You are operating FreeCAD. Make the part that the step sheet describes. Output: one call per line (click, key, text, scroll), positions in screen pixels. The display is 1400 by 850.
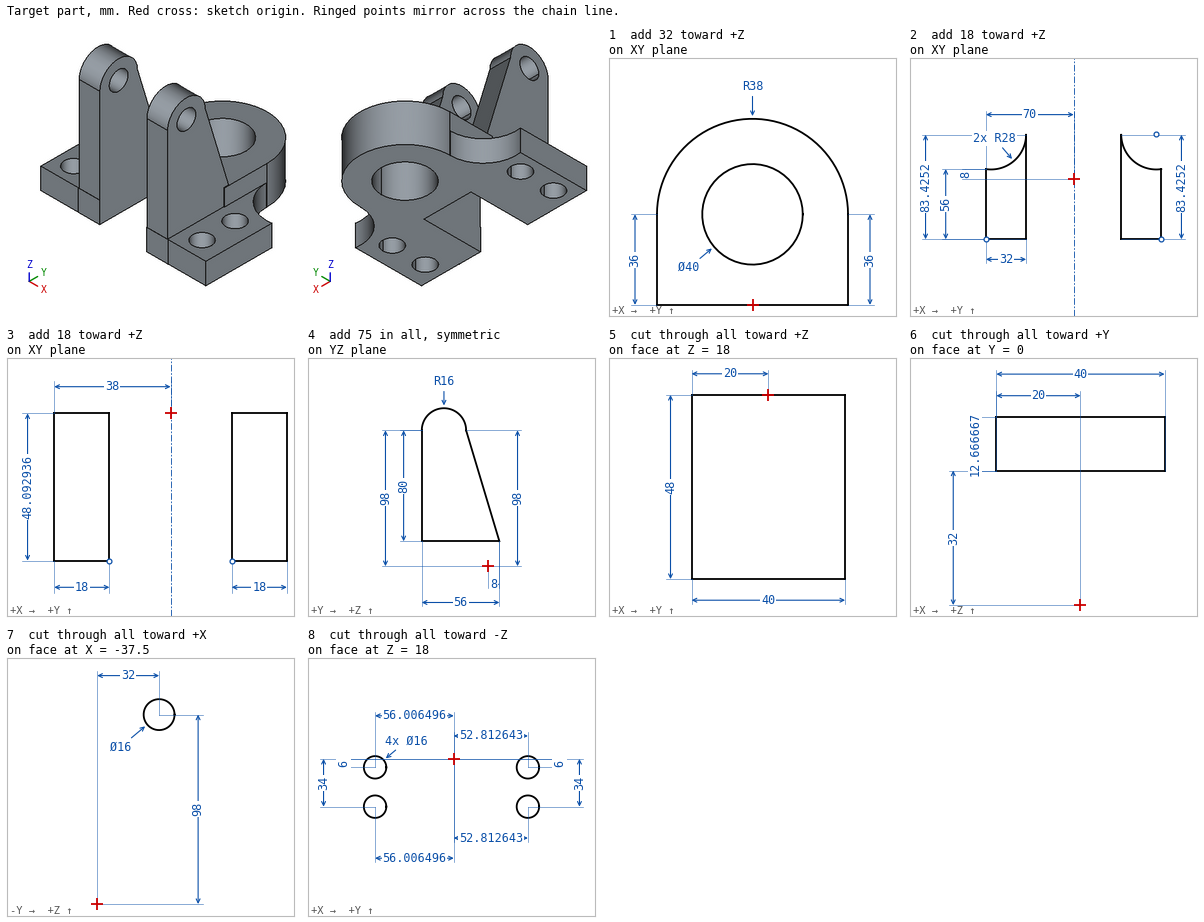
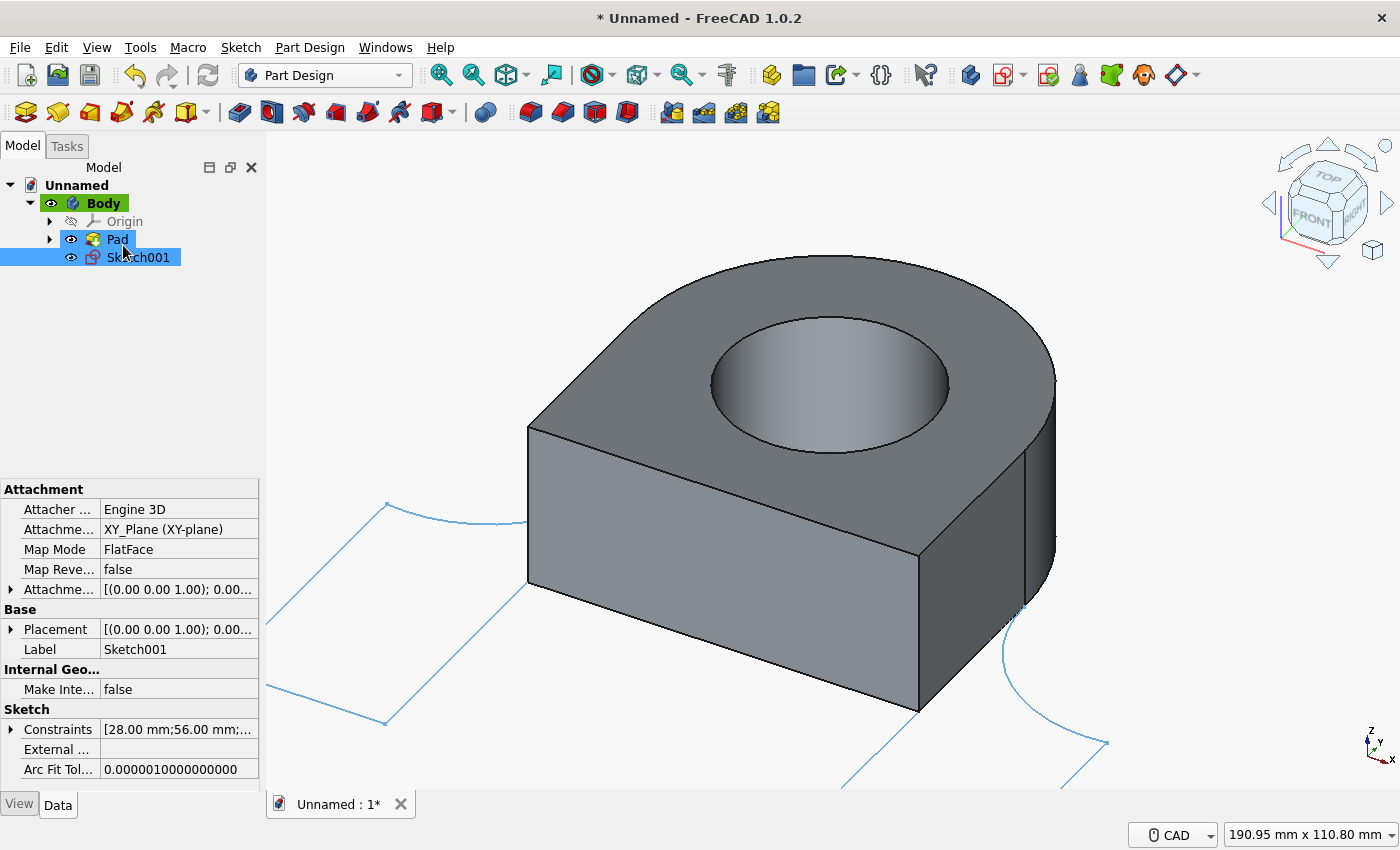
click(26, 112)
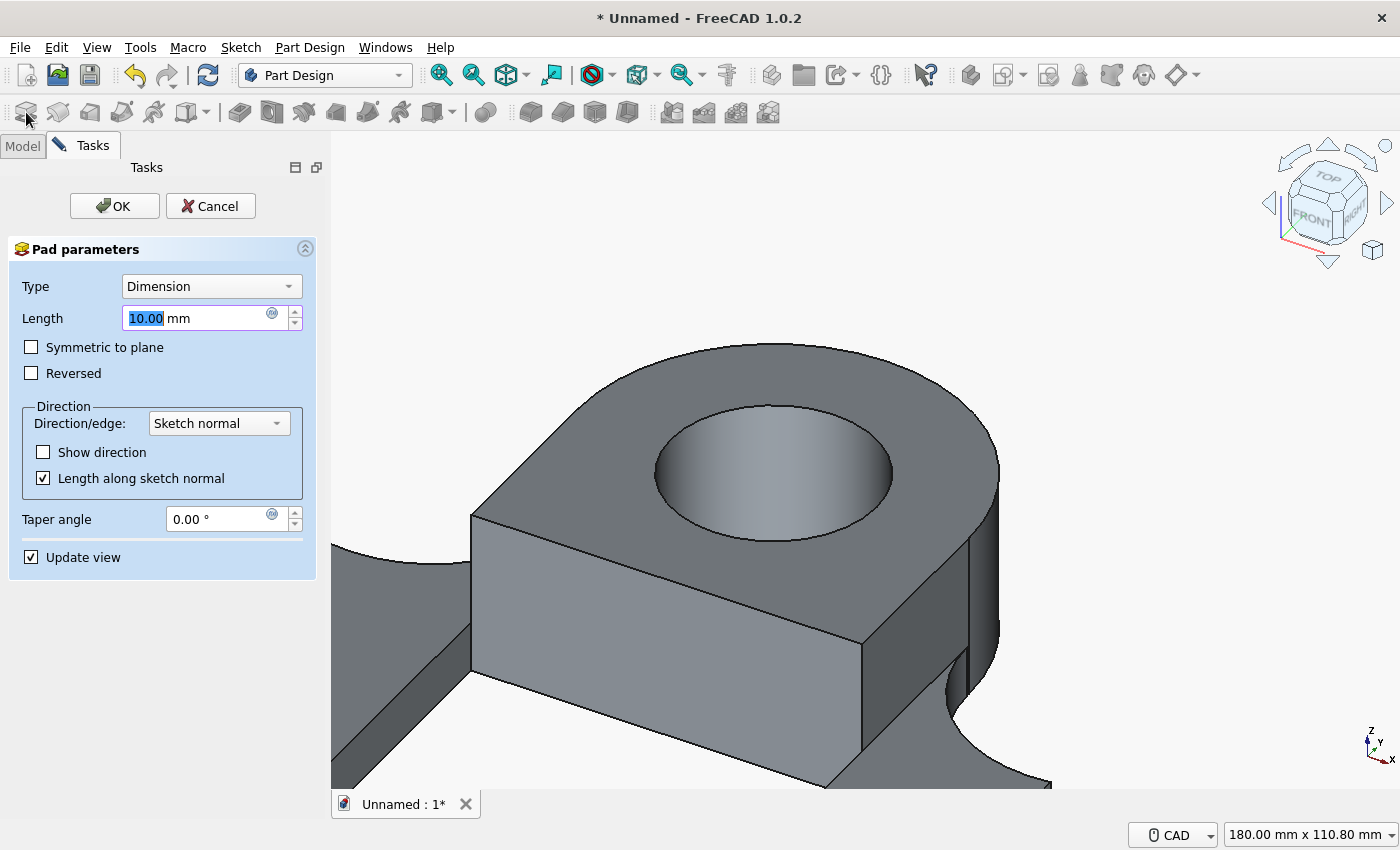
text(18)
key(Tab)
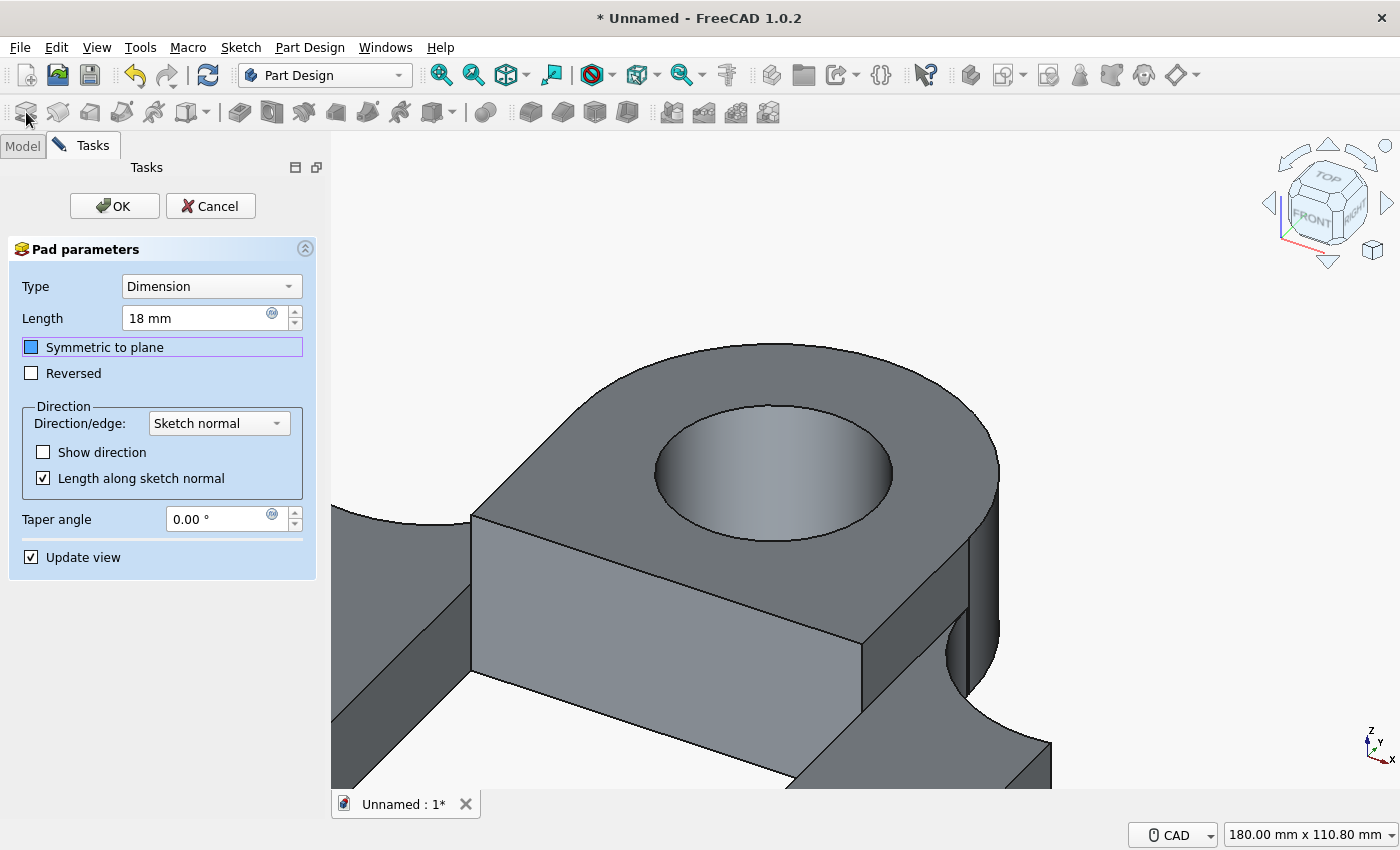
click(115, 206)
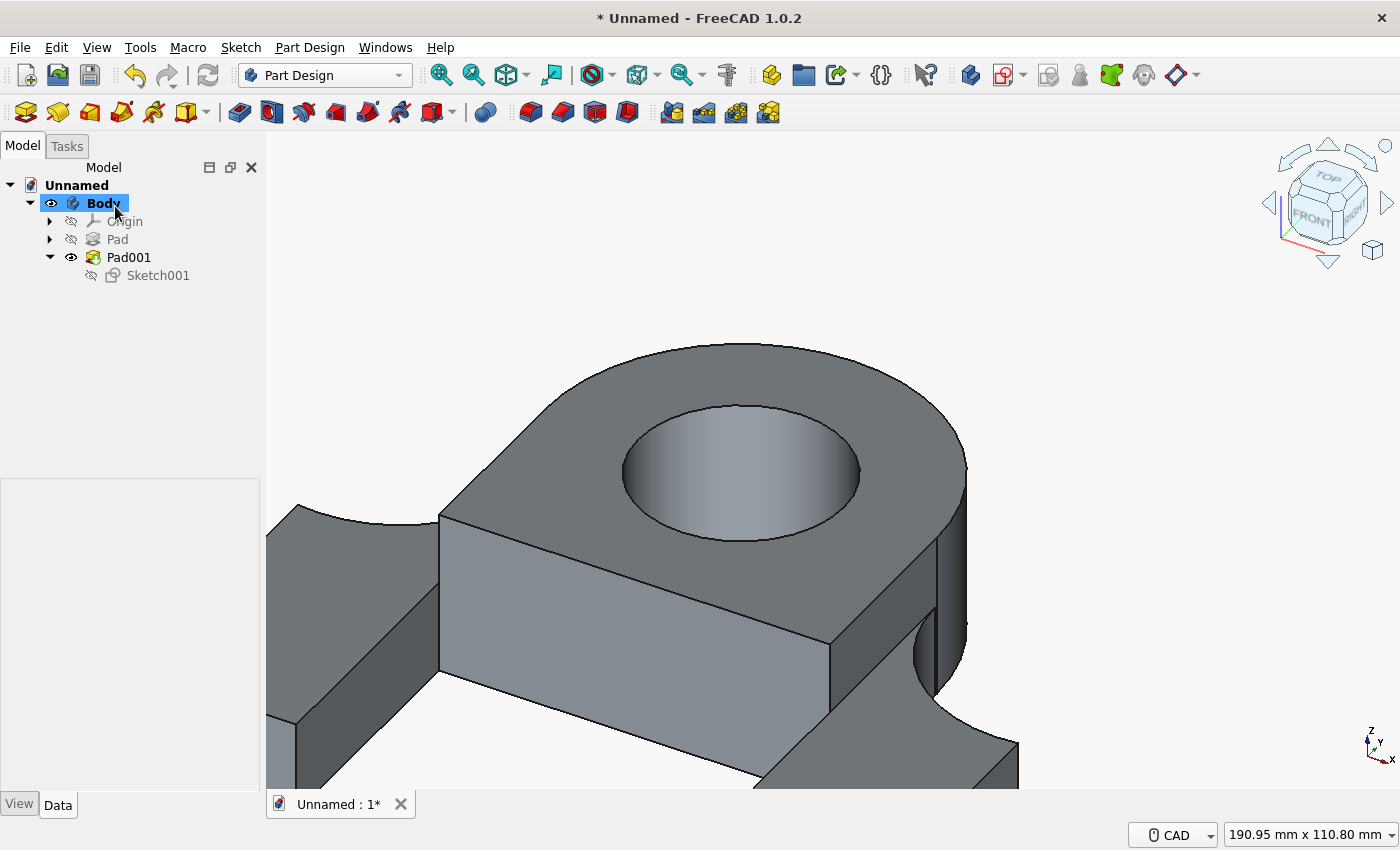
click(442, 76)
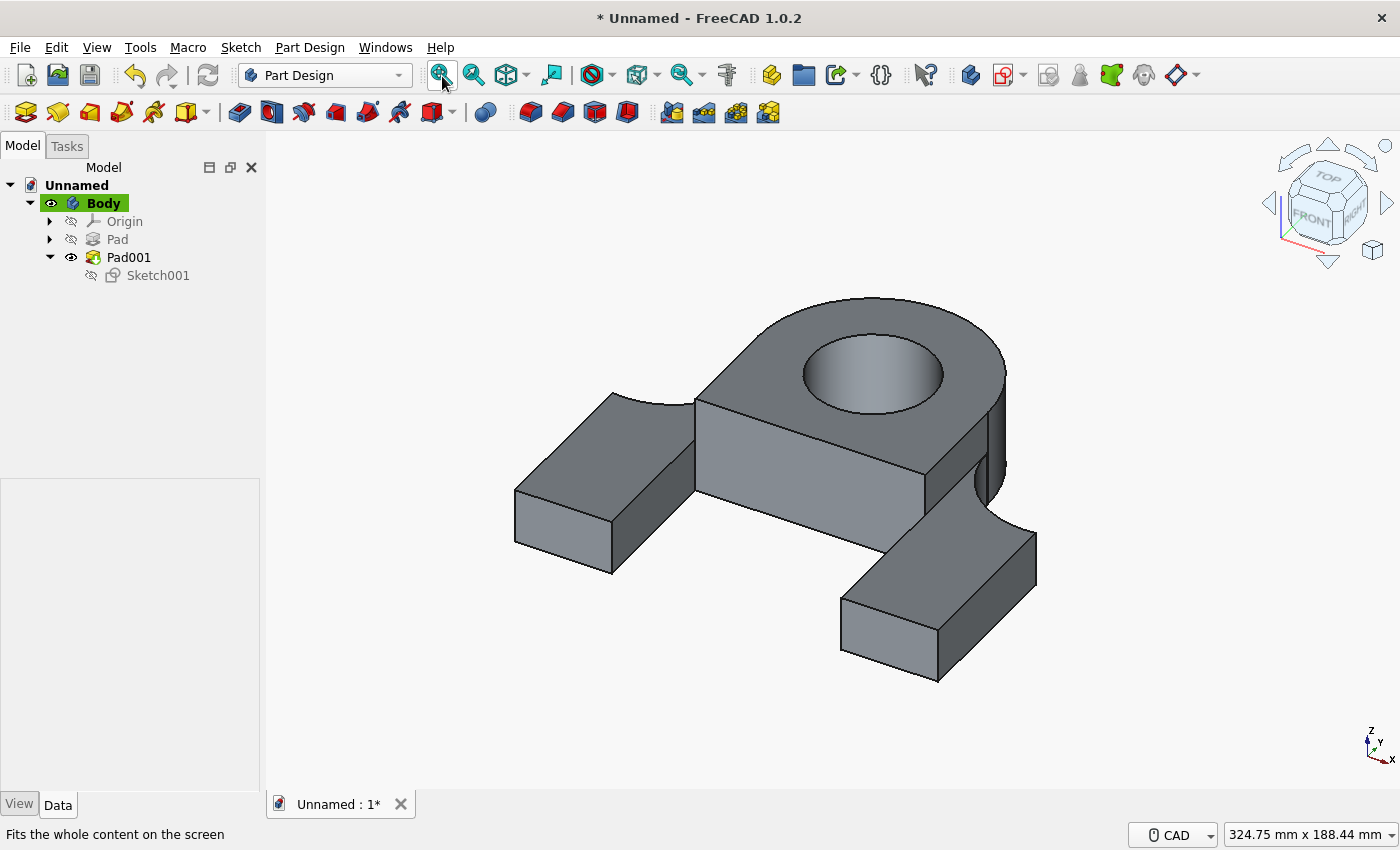
click(1004, 76)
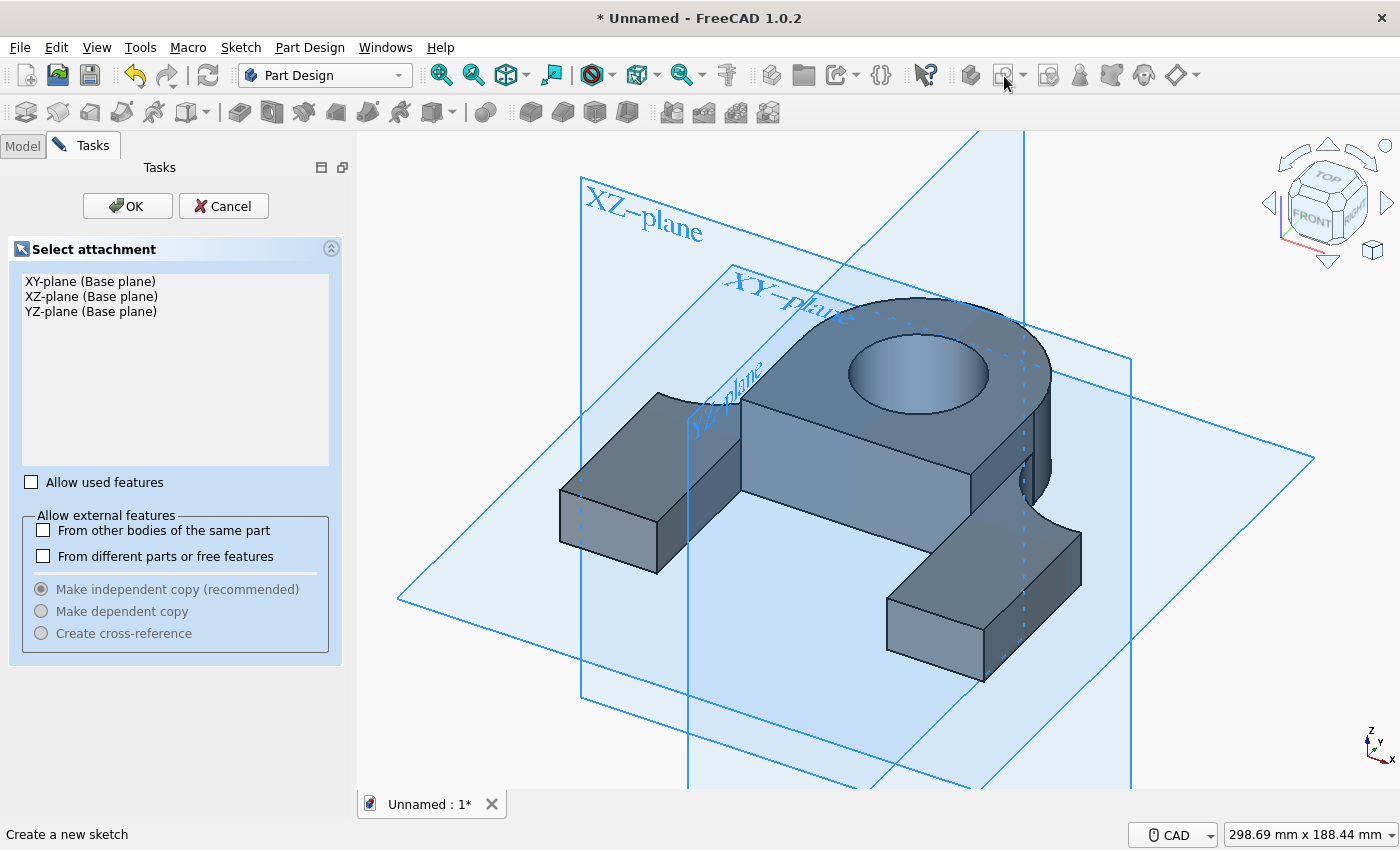
click(82, 282)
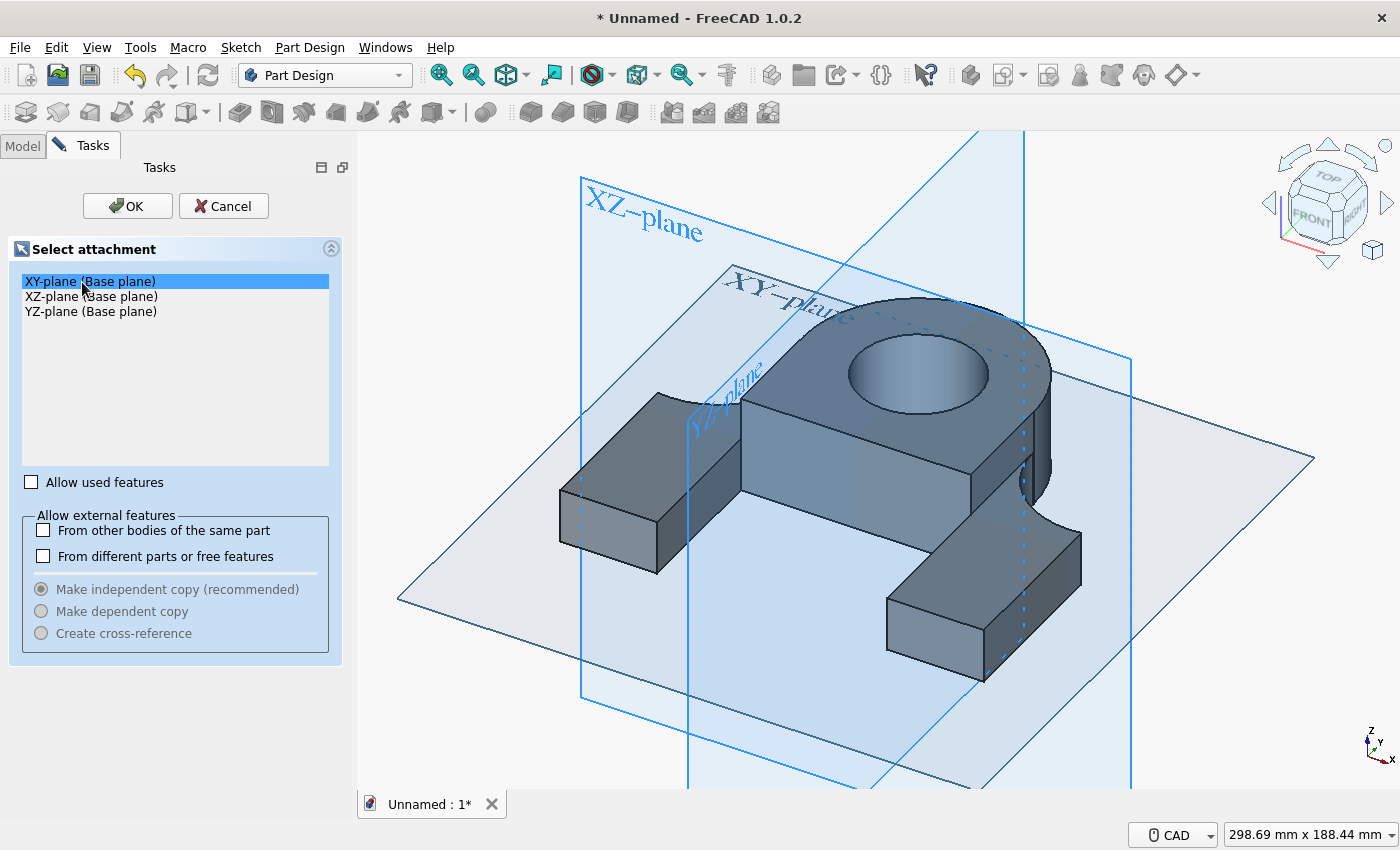
click(128, 206)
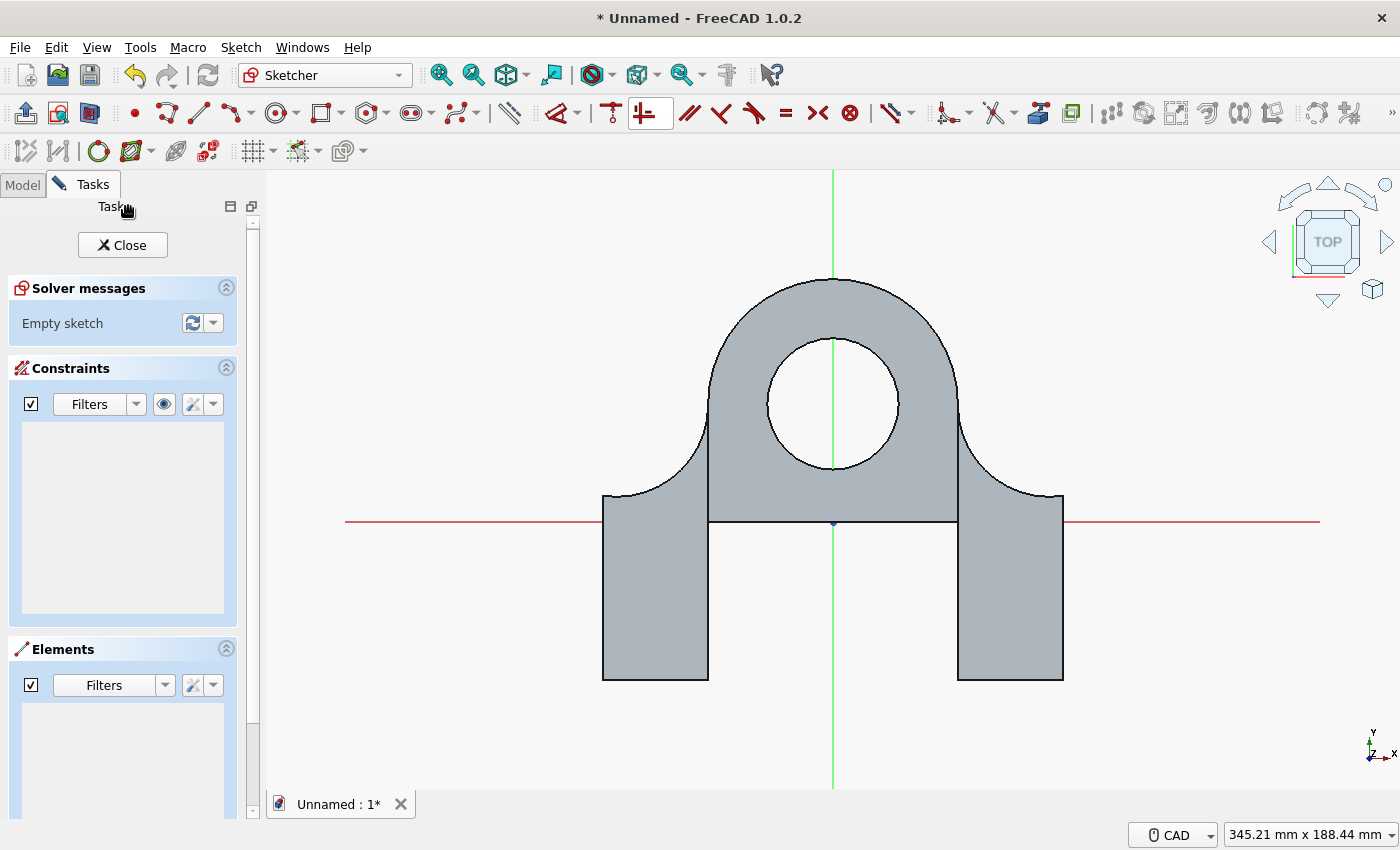
click(90, 114)